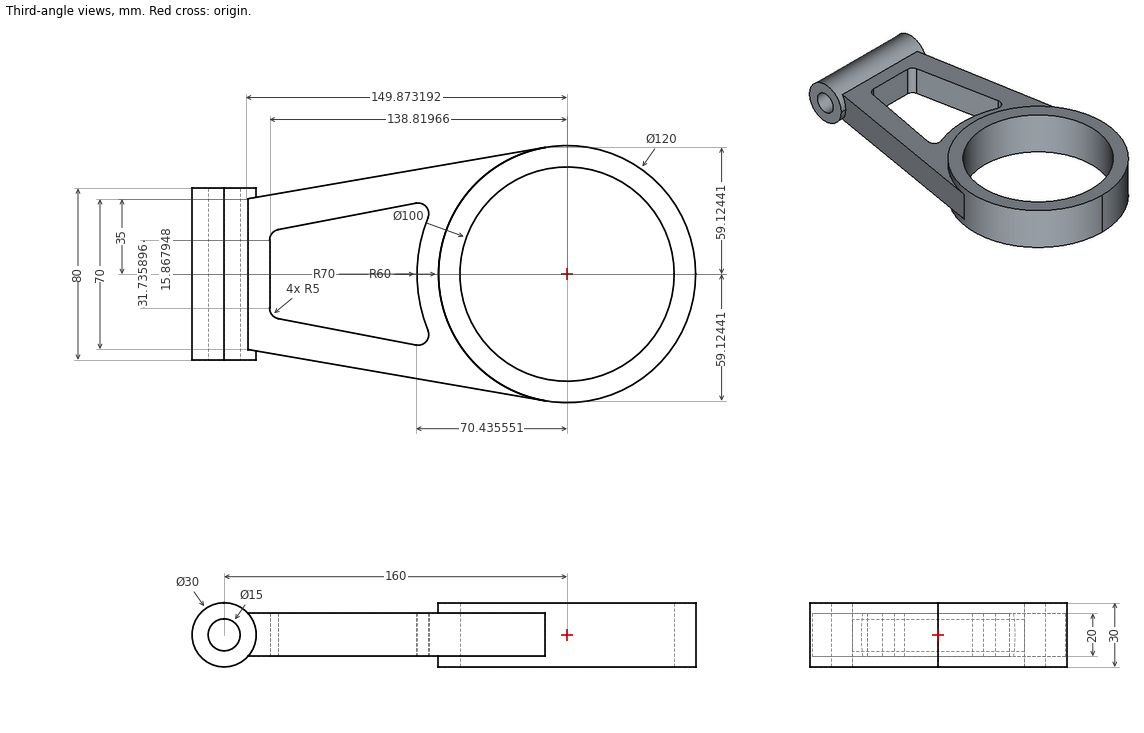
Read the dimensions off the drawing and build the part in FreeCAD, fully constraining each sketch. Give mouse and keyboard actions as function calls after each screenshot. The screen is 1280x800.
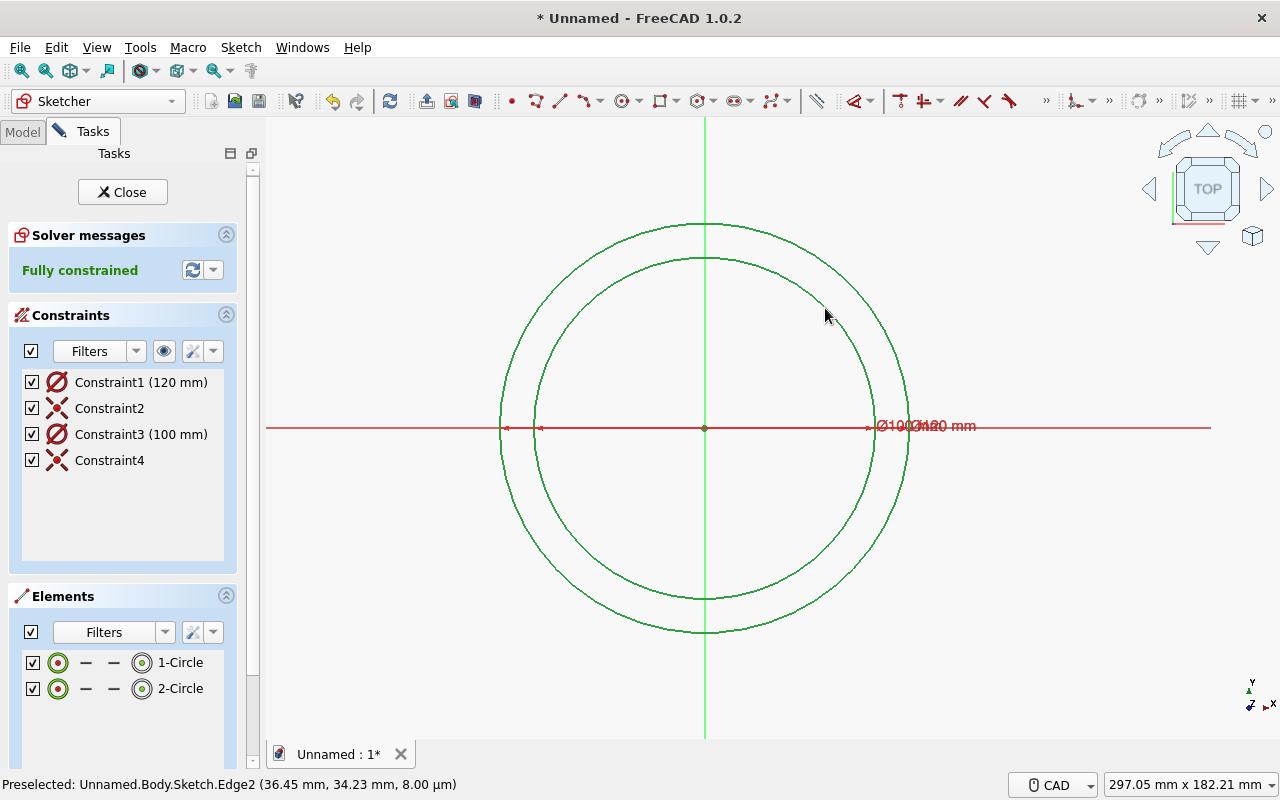
click(123, 192)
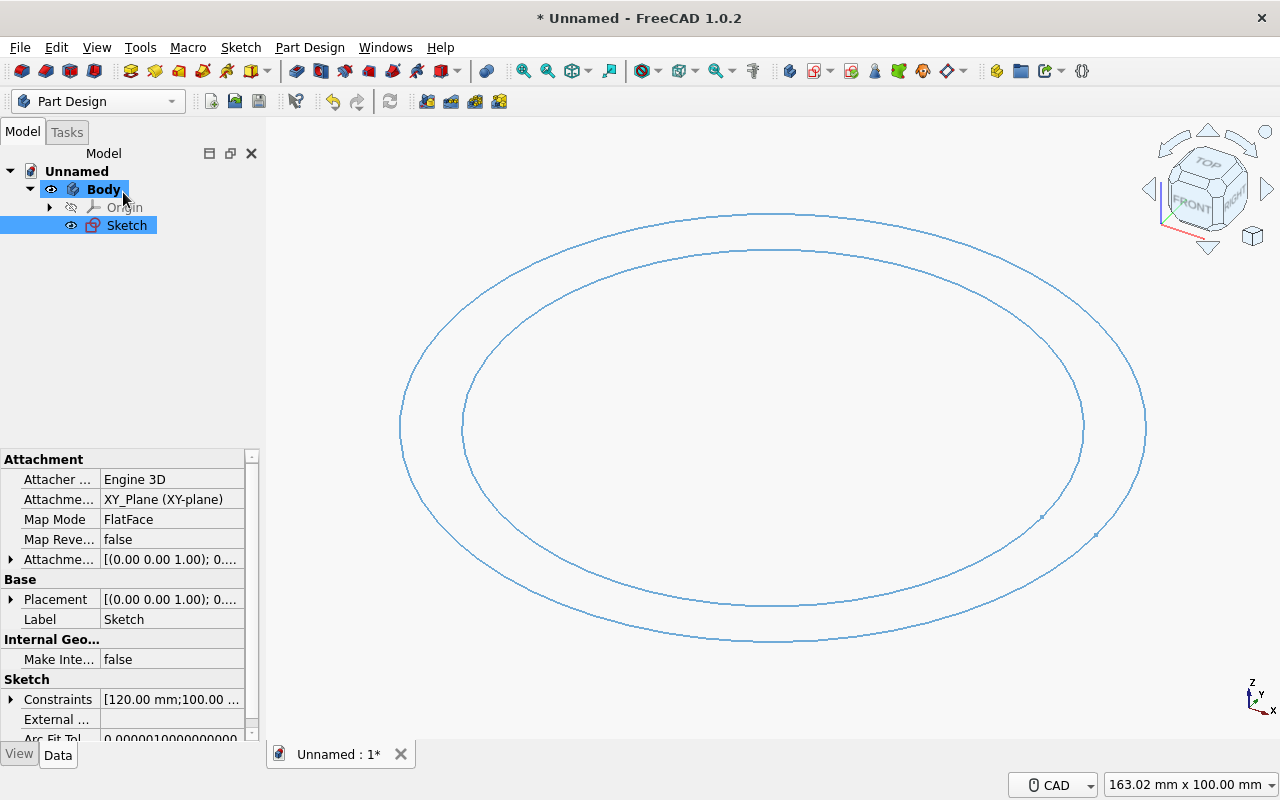
click(132, 72)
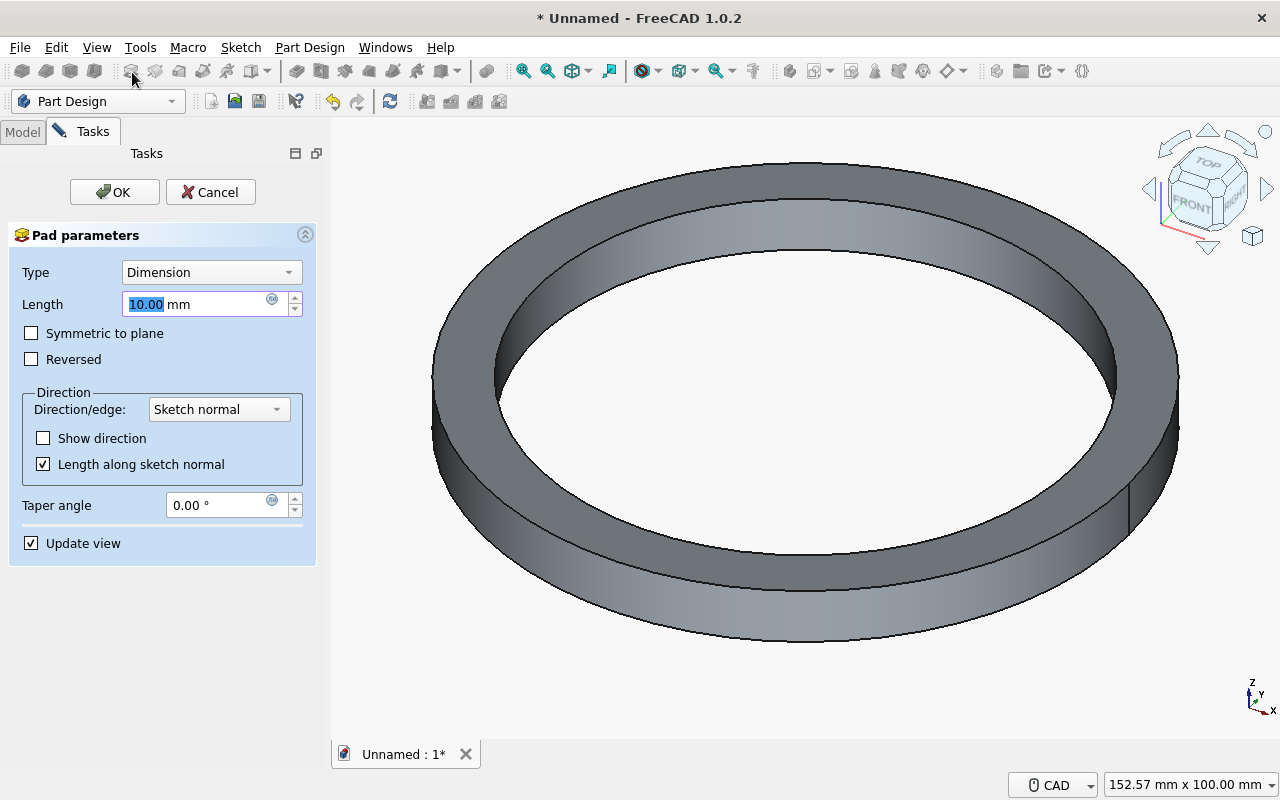
text(30)
key(Tab)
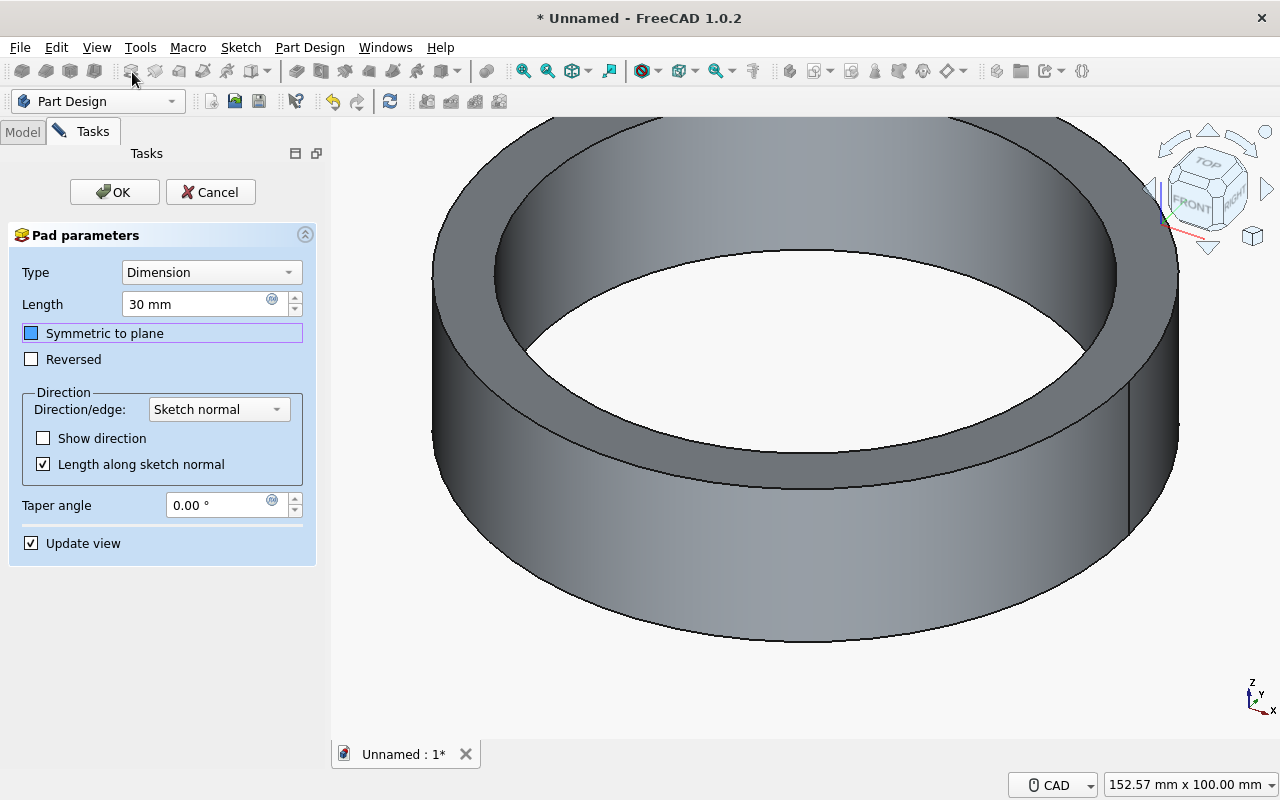
click(30, 333)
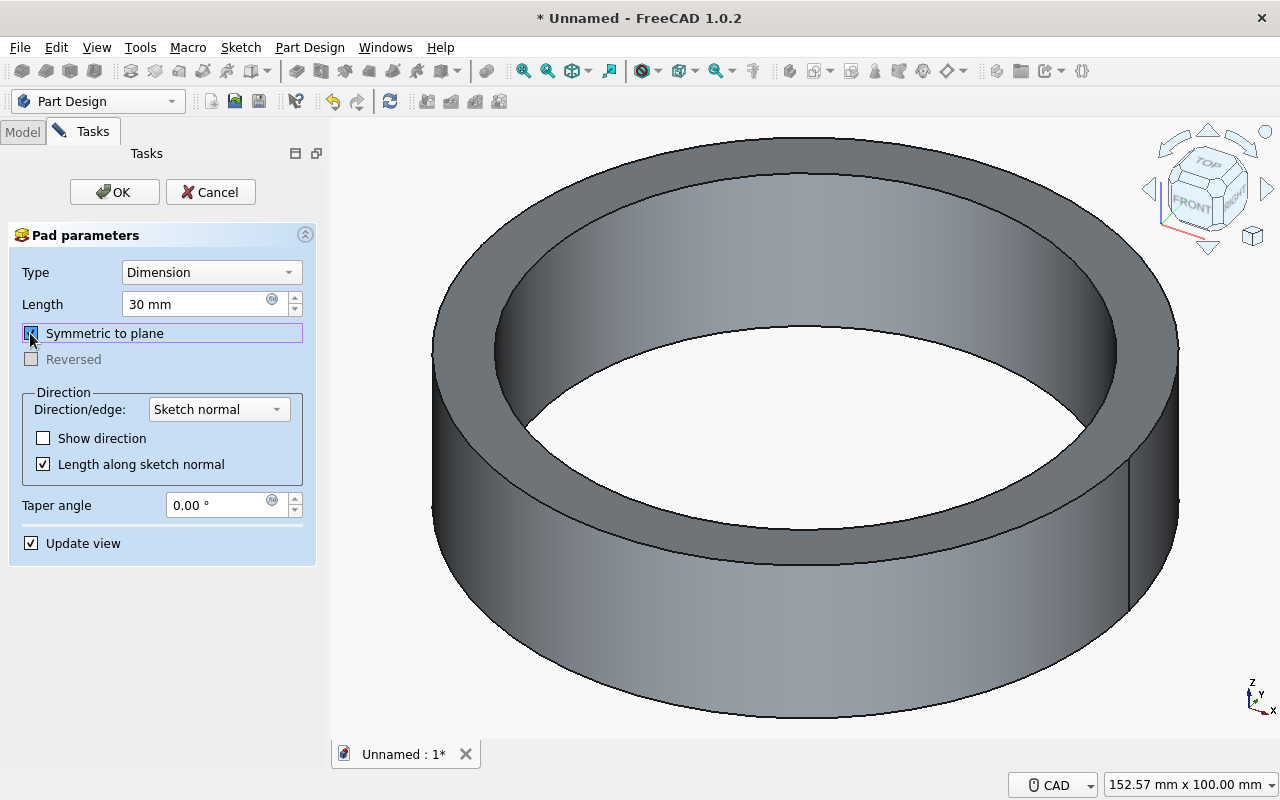
click(115, 192)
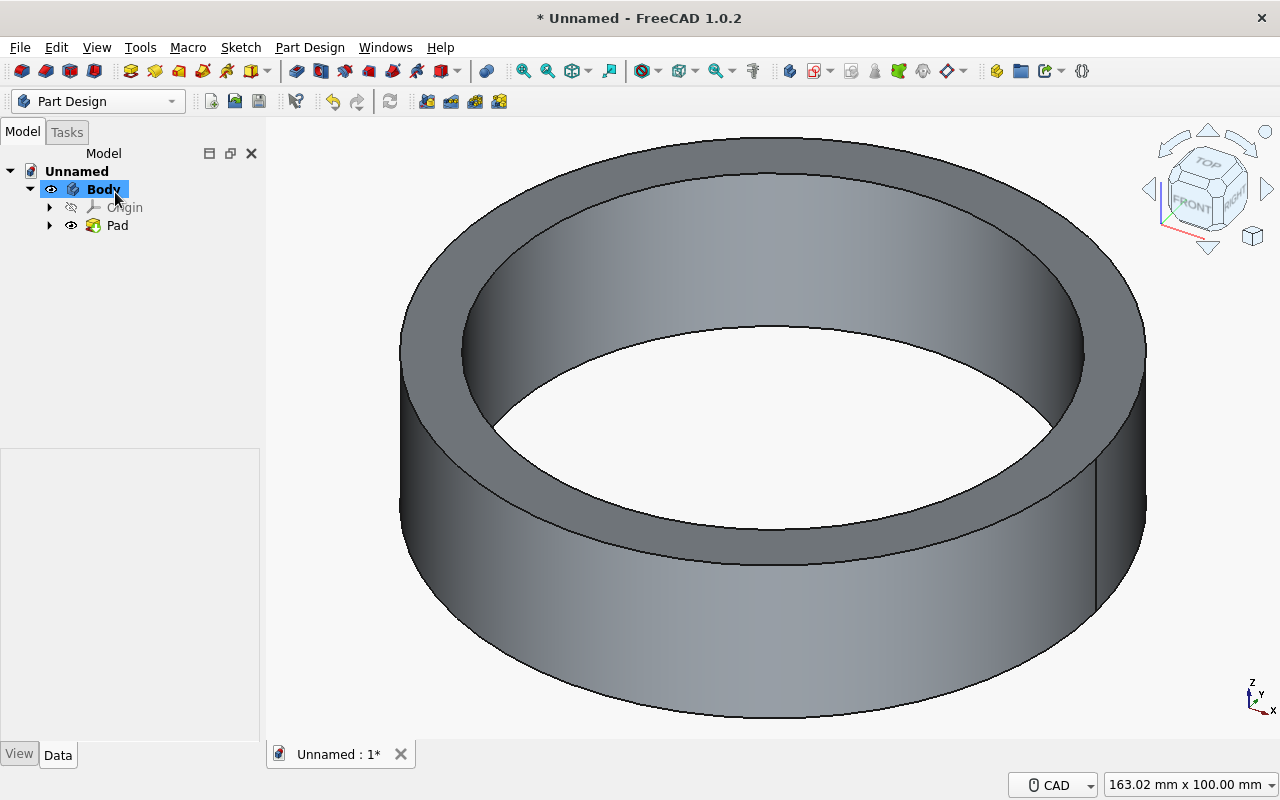
click(524, 72)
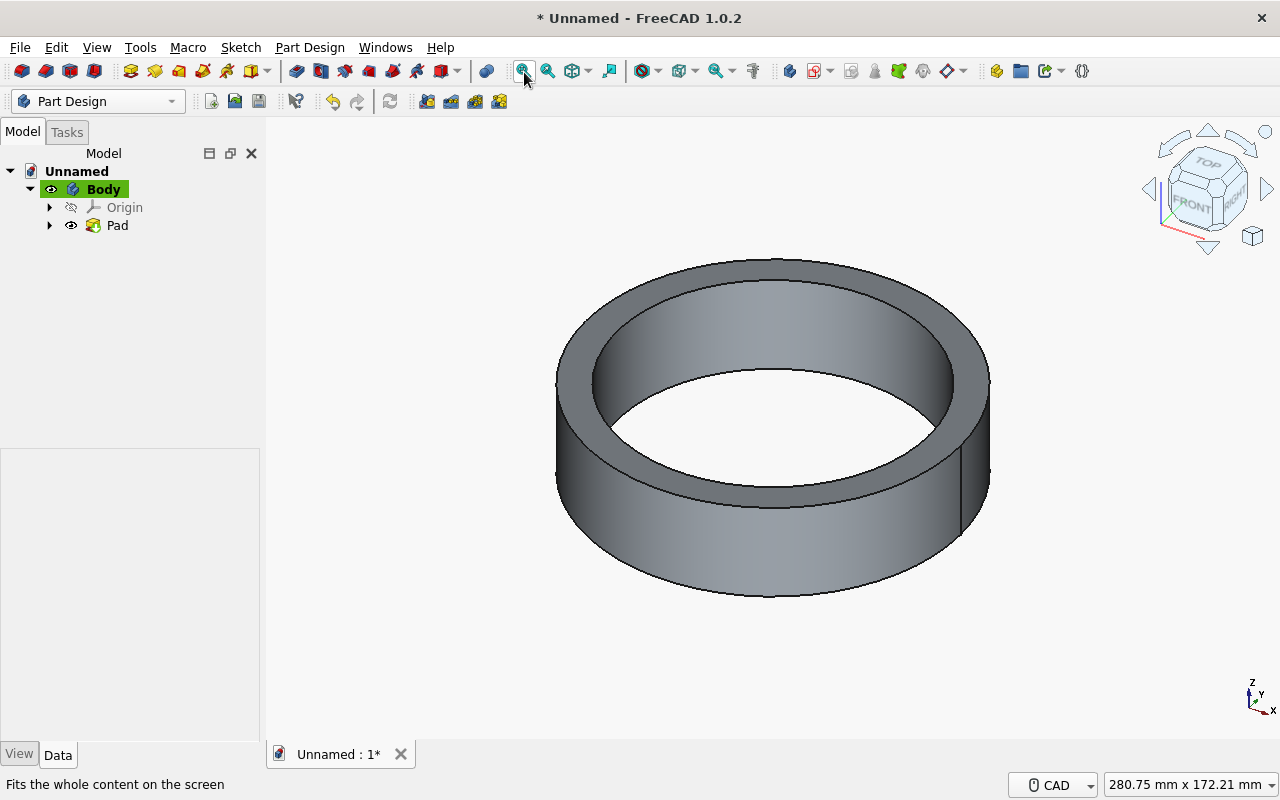
click(790, 72)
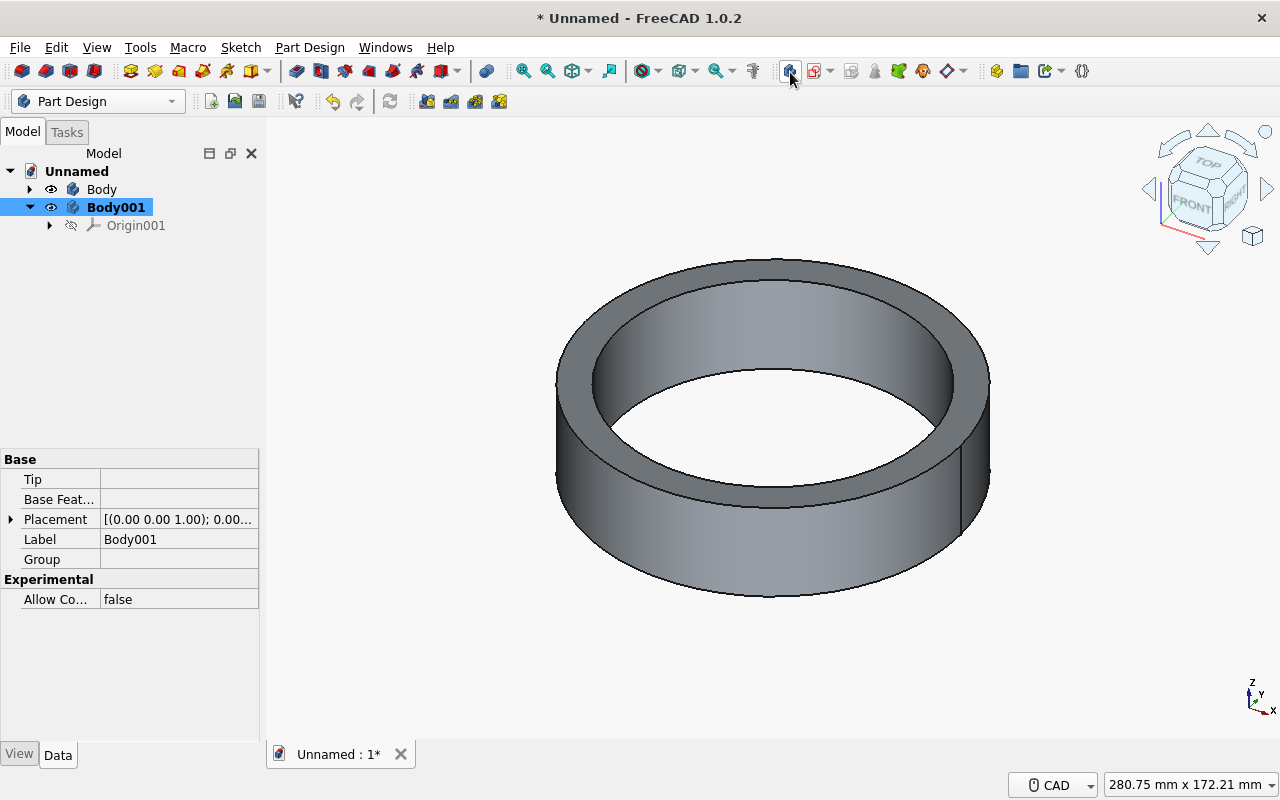
click(306, 699)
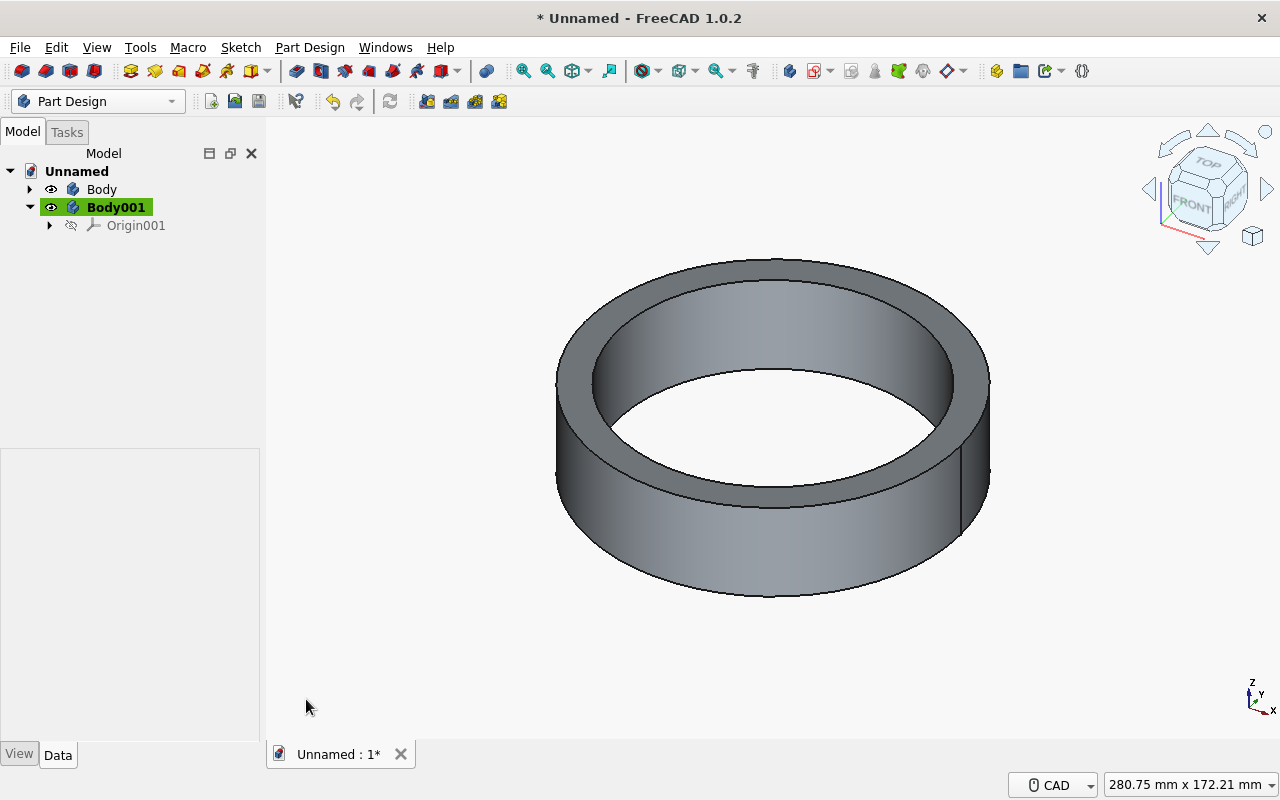
click(814, 72)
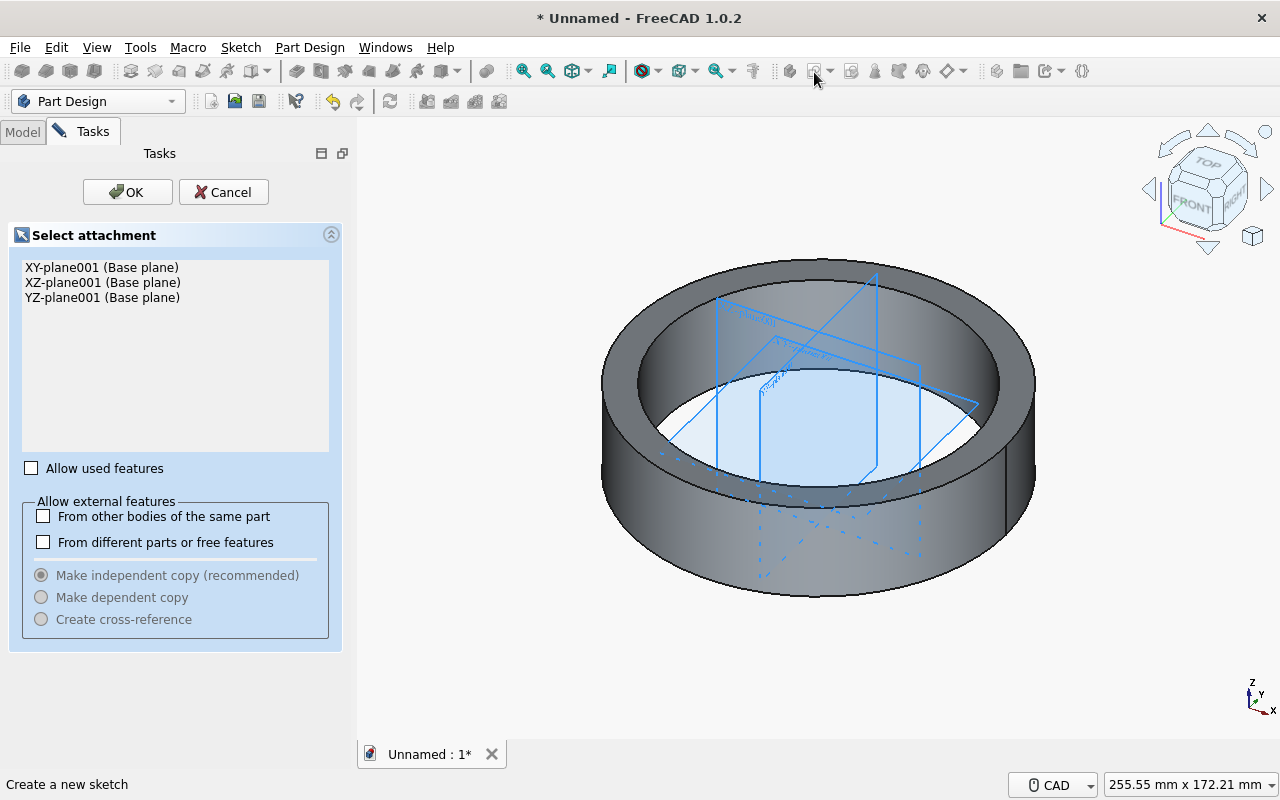
click(82, 282)